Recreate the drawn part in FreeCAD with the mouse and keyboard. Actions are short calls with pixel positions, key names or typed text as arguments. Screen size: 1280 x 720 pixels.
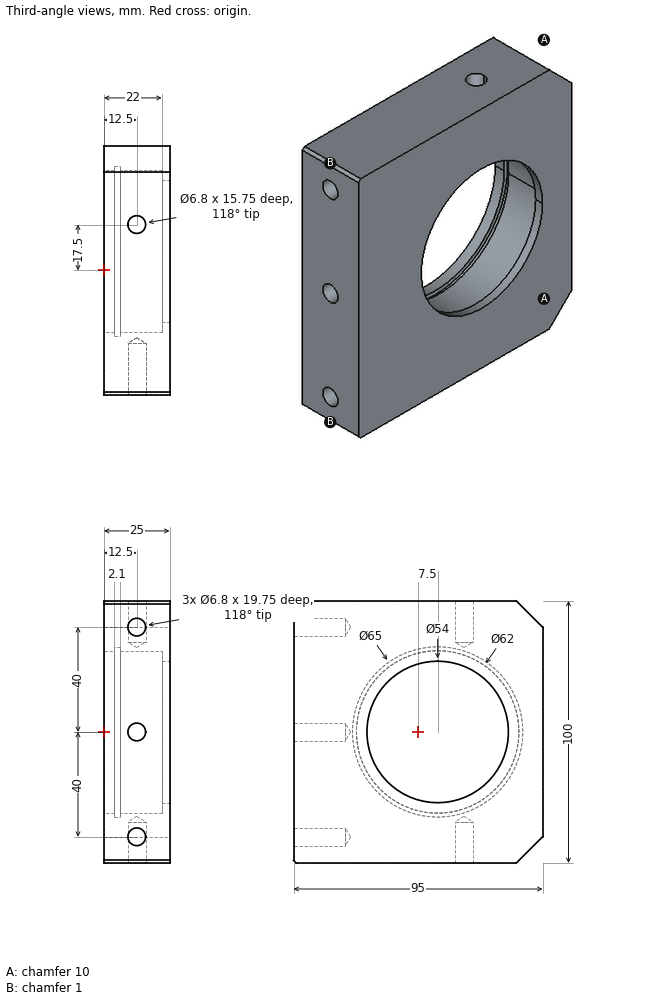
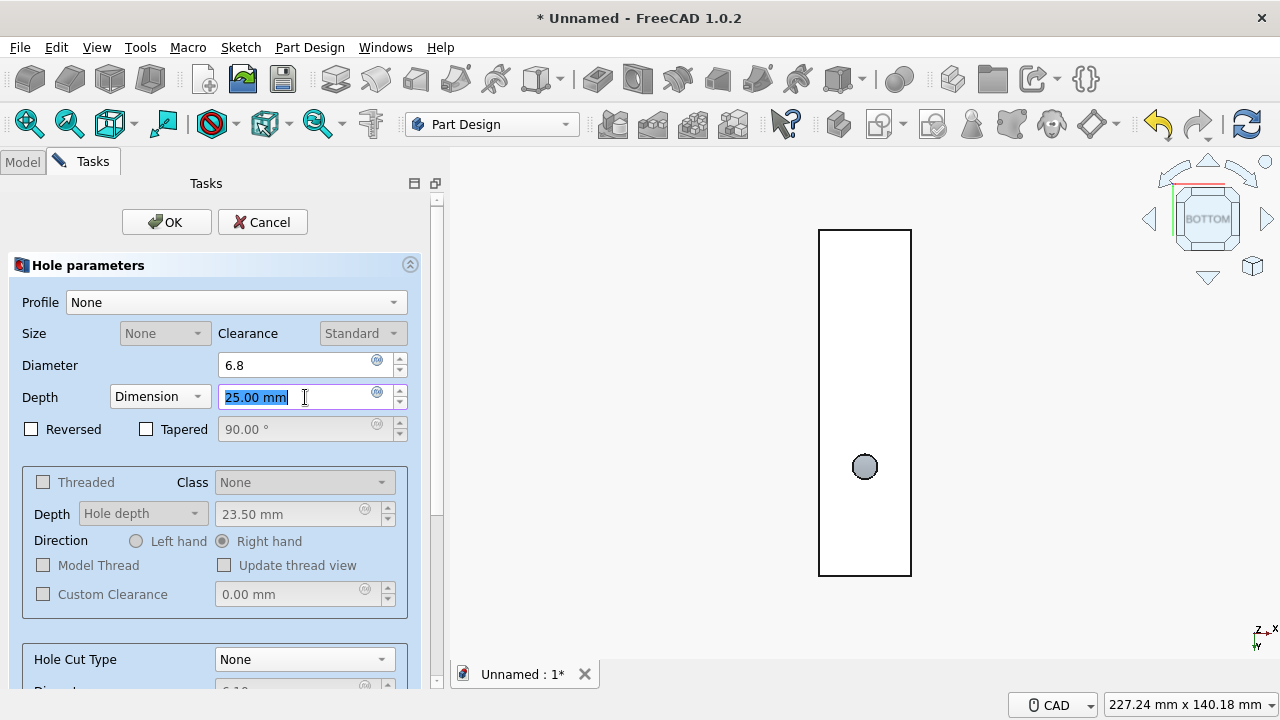
text(15.75)
key(Tab)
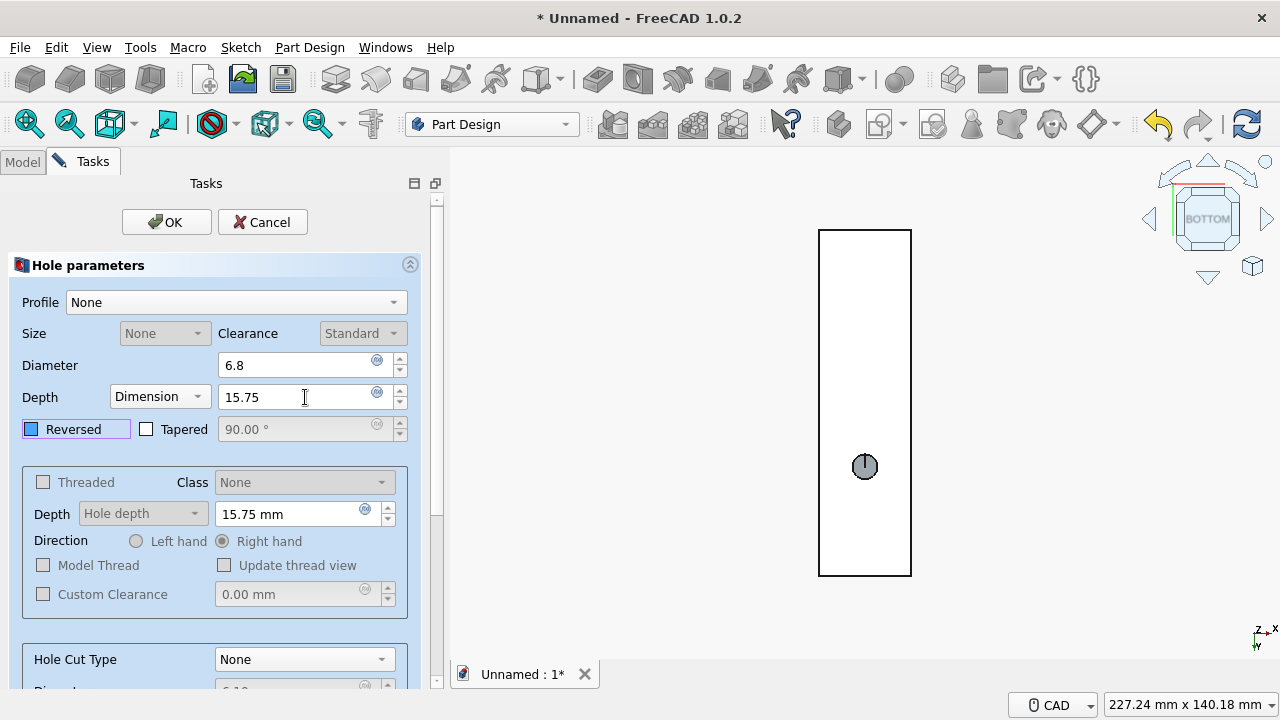
click(167, 222)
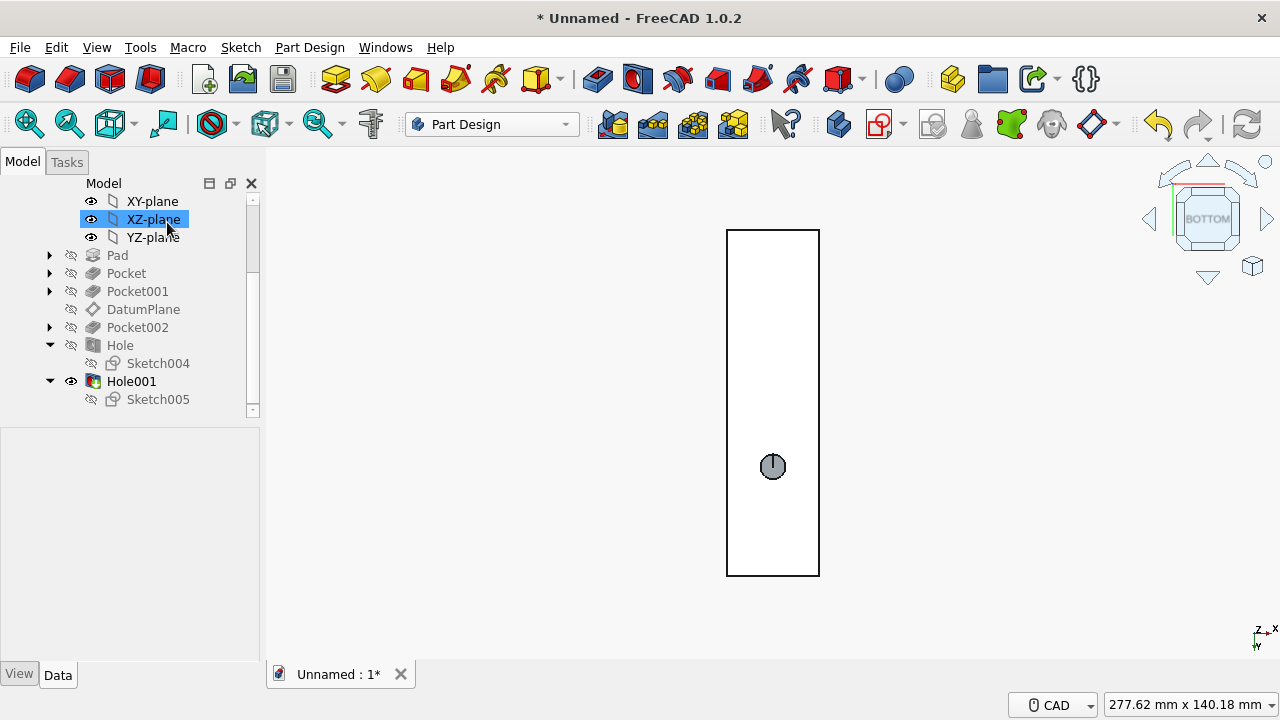
click(773, 575)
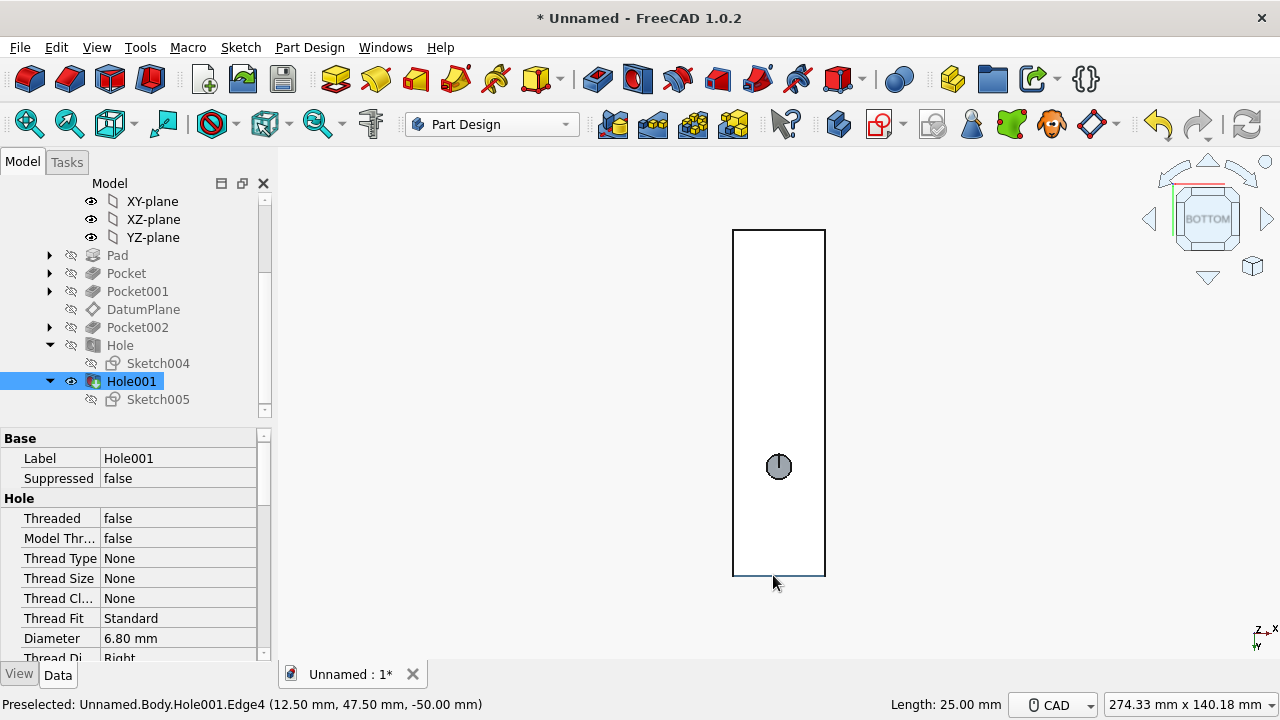
key(0)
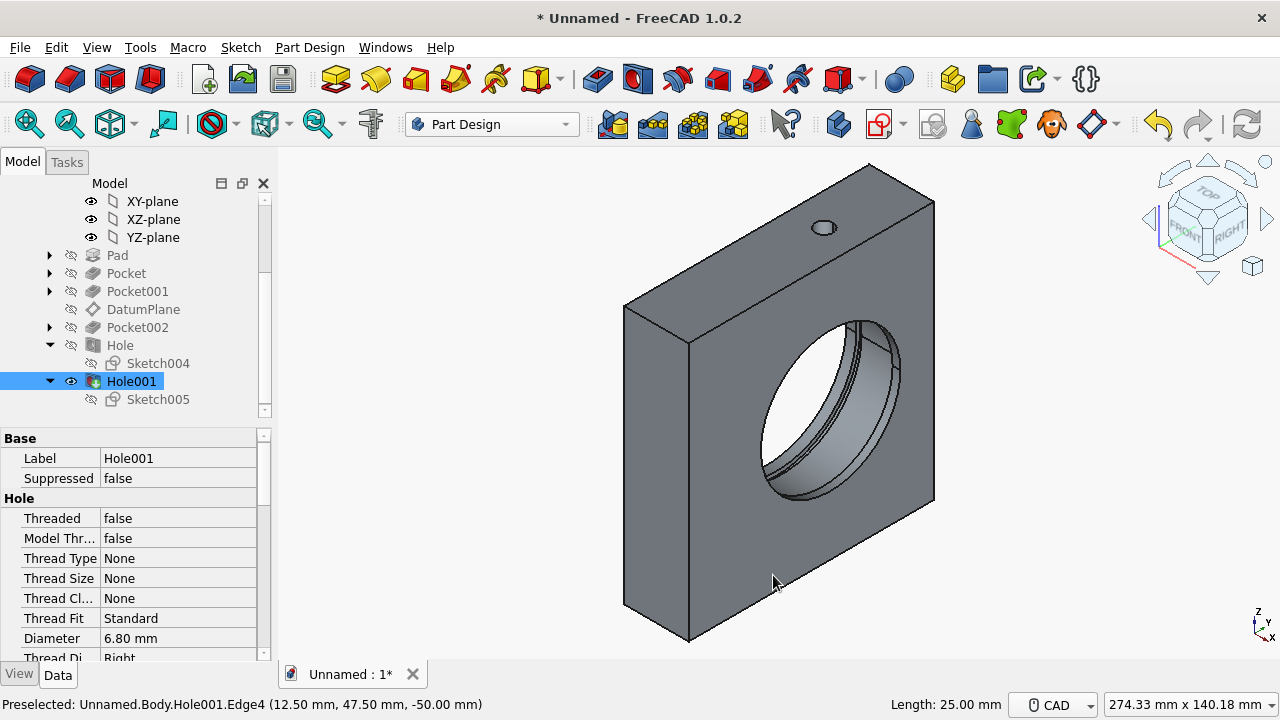
key(2)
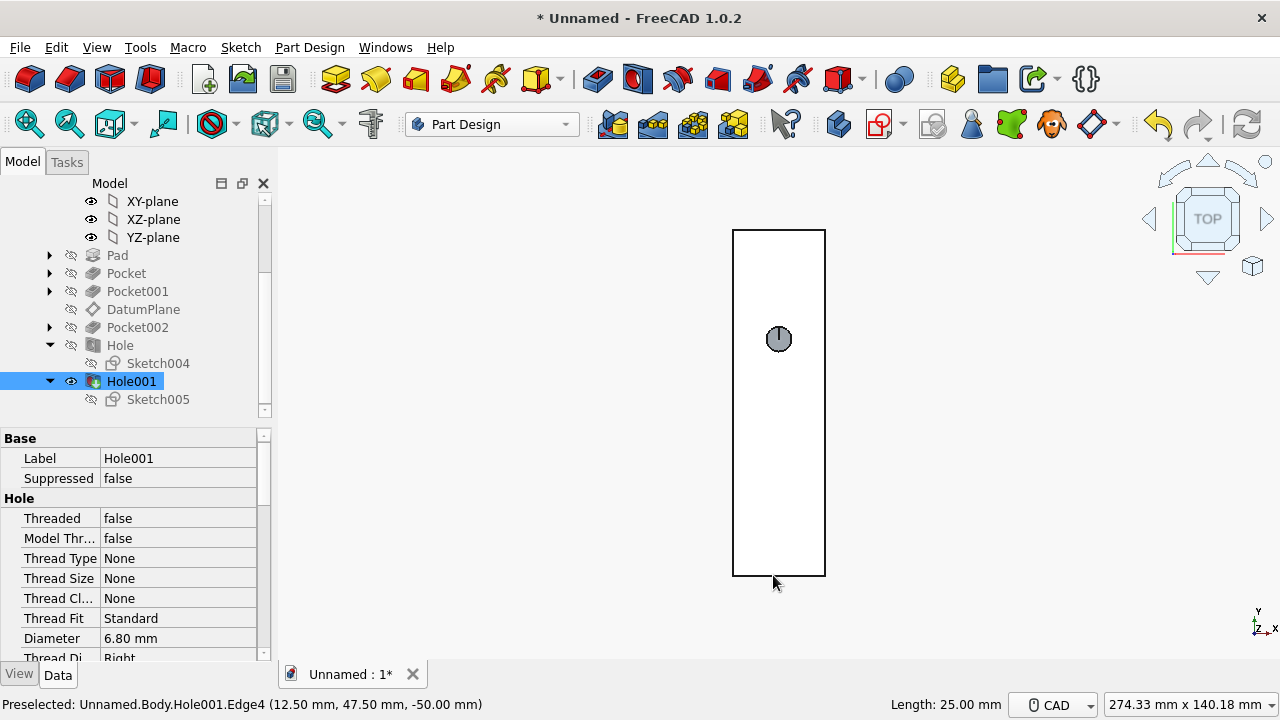
click(779, 229, ctrl)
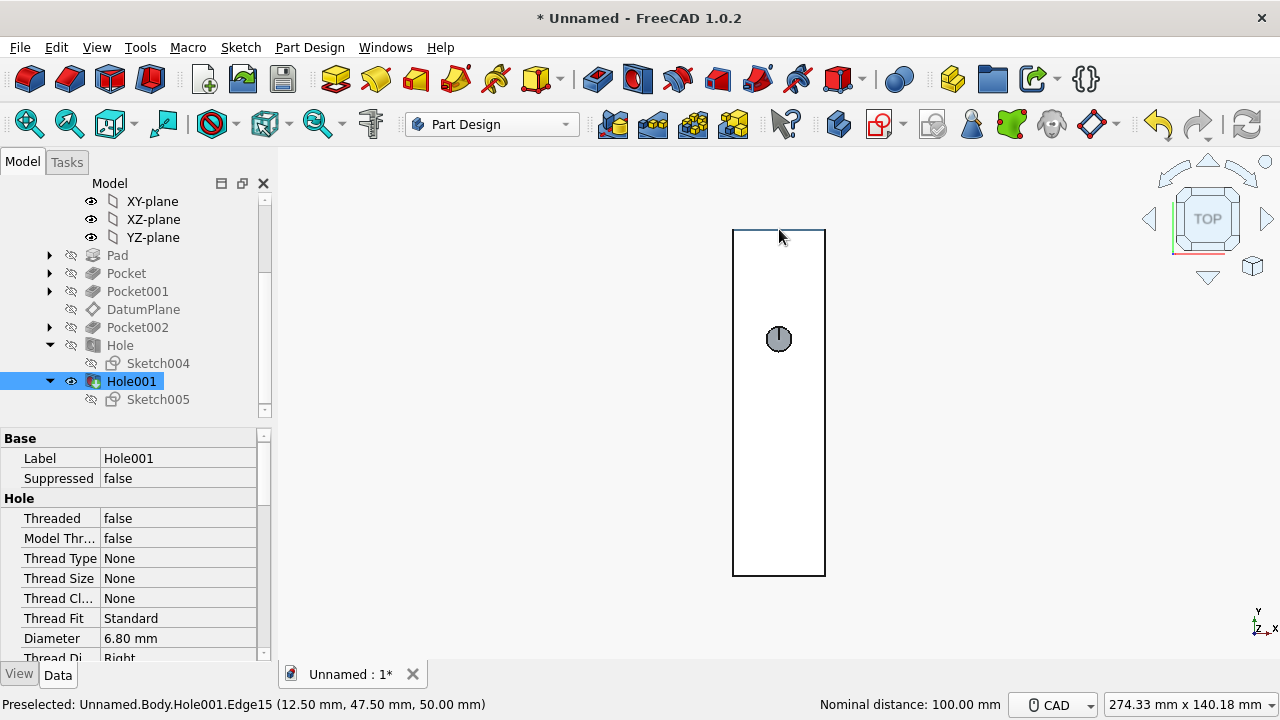
click(70, 80)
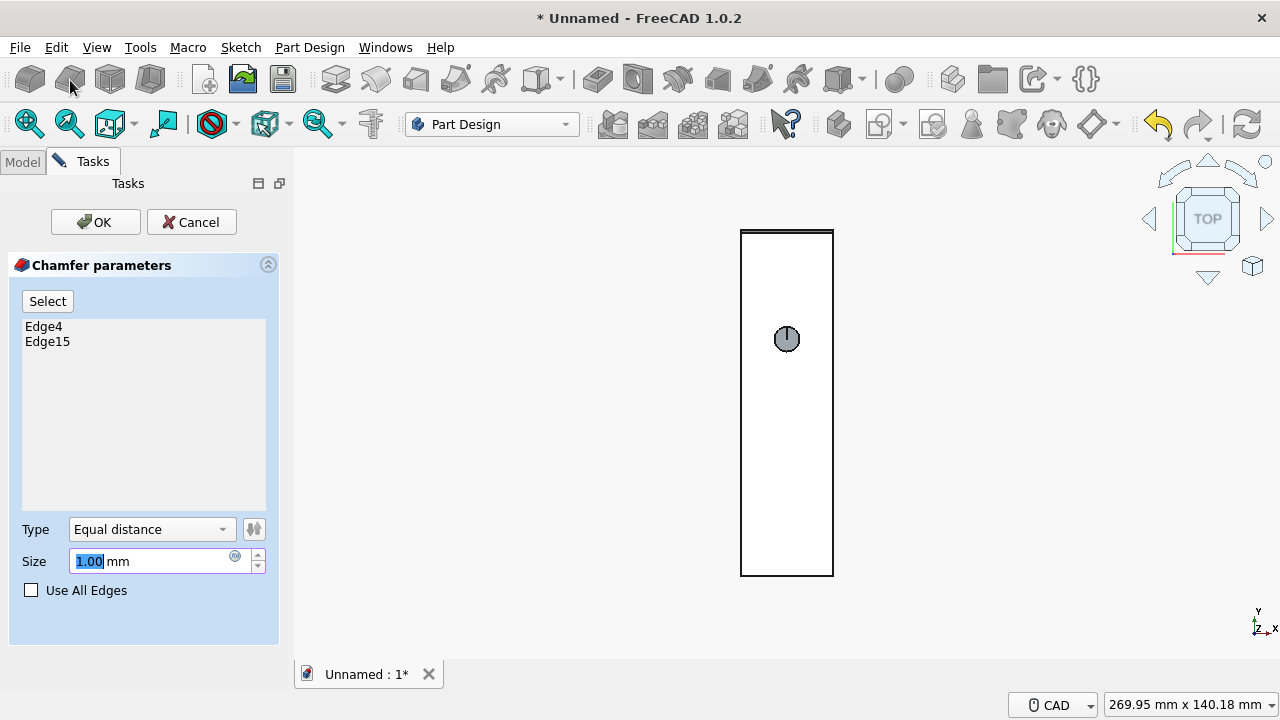
text(10)
key(Tab)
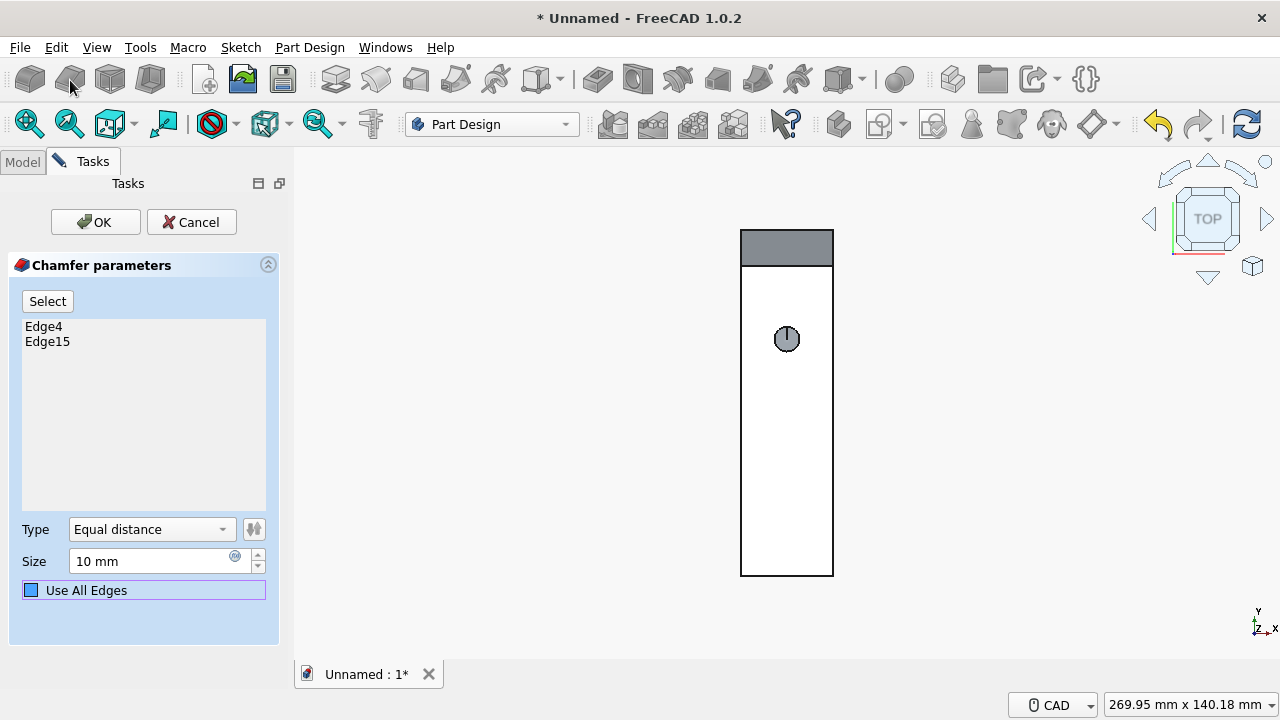
click(96, 222)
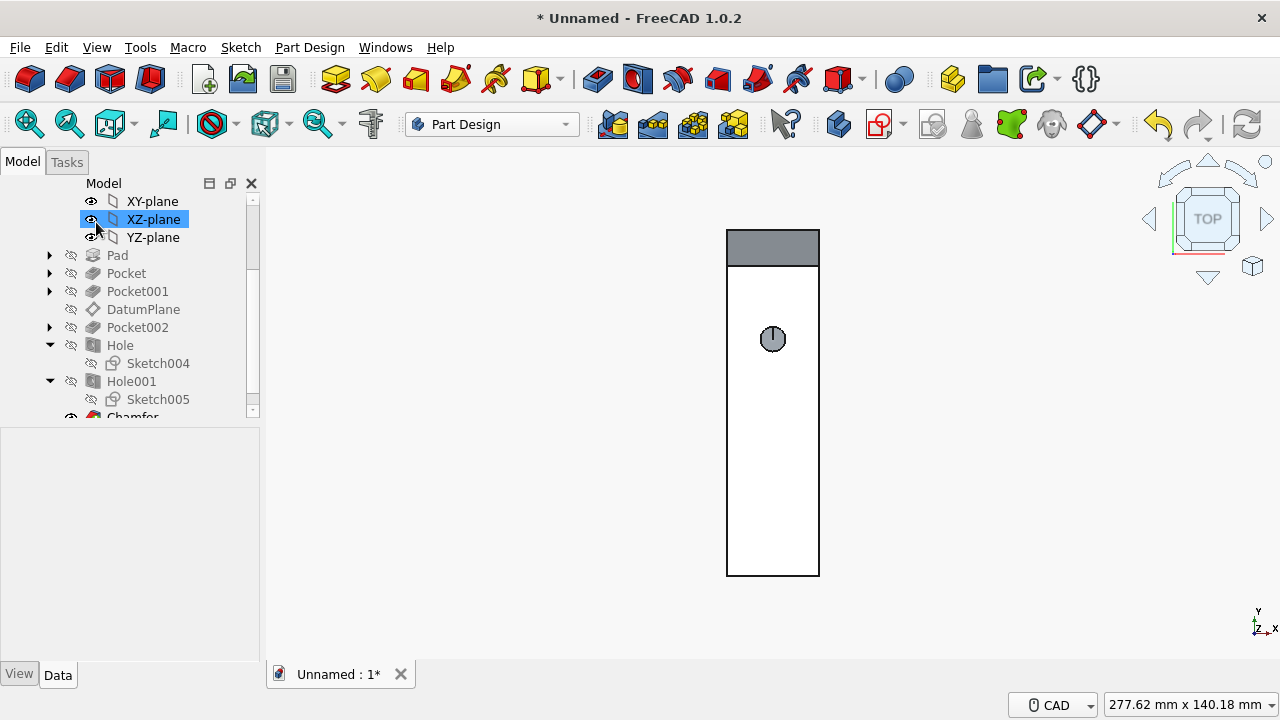
click(773, 575)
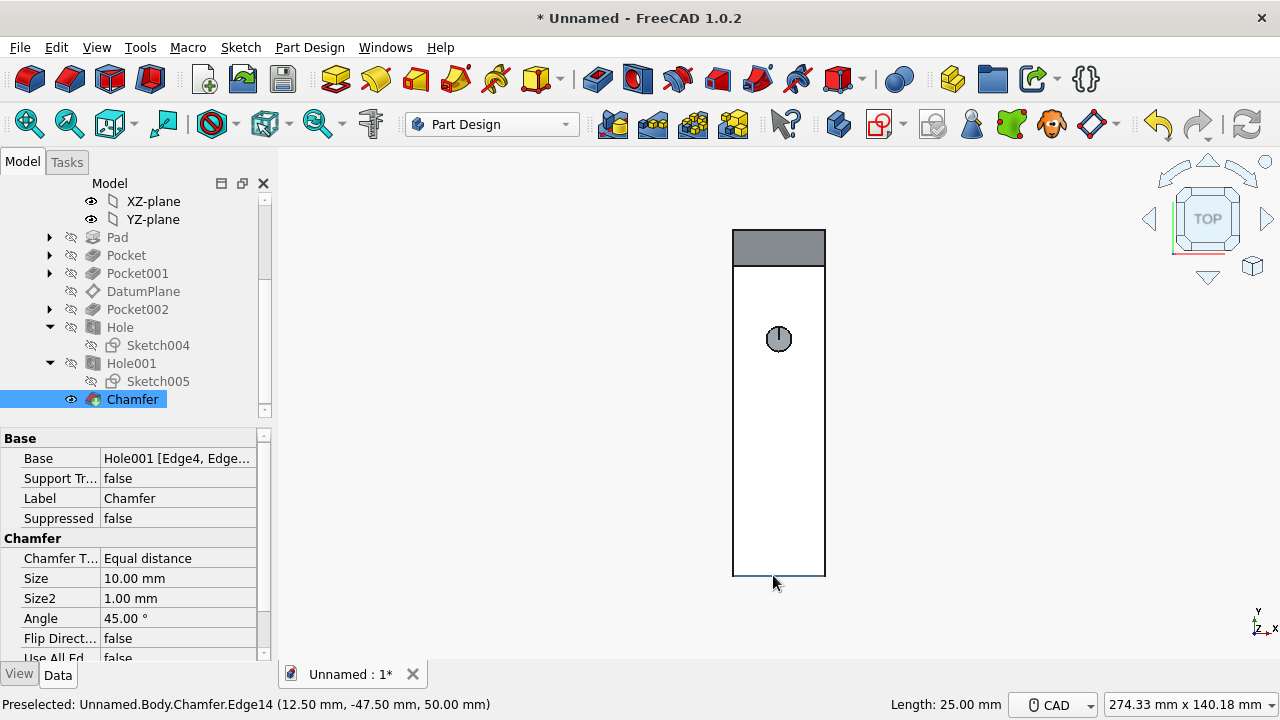
key(0)